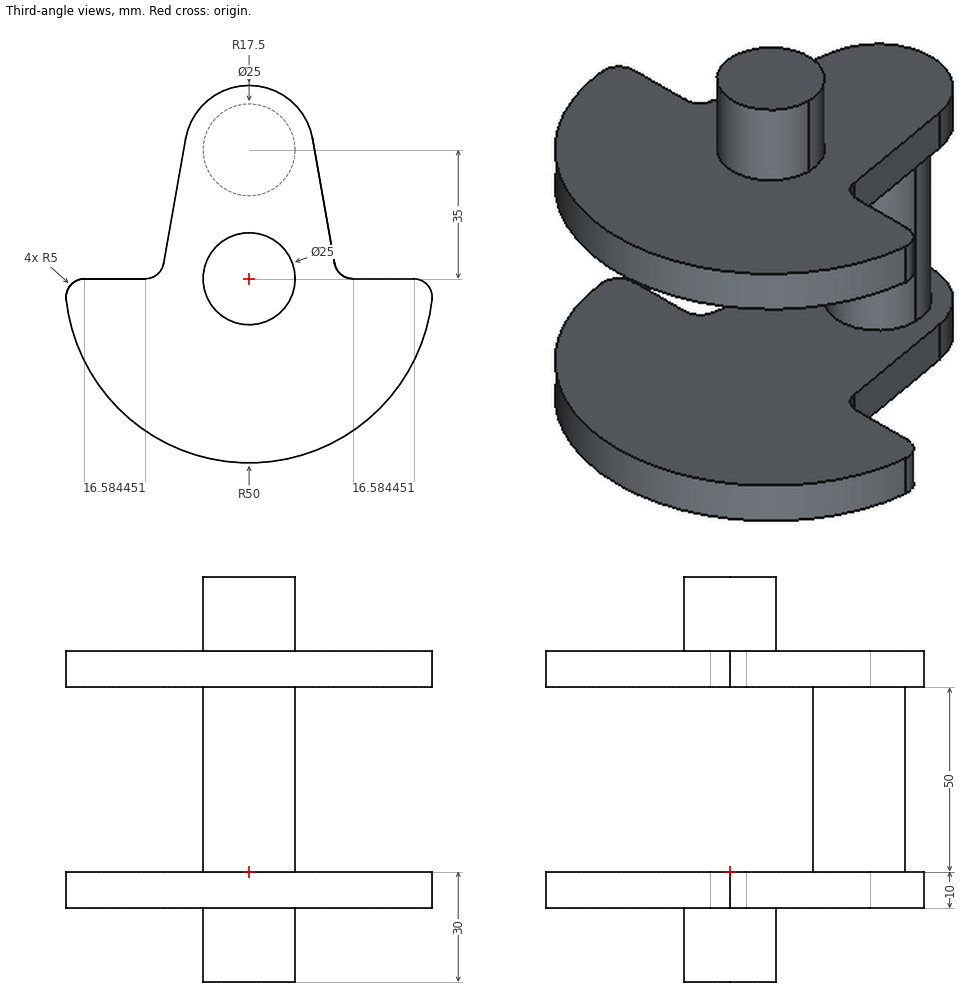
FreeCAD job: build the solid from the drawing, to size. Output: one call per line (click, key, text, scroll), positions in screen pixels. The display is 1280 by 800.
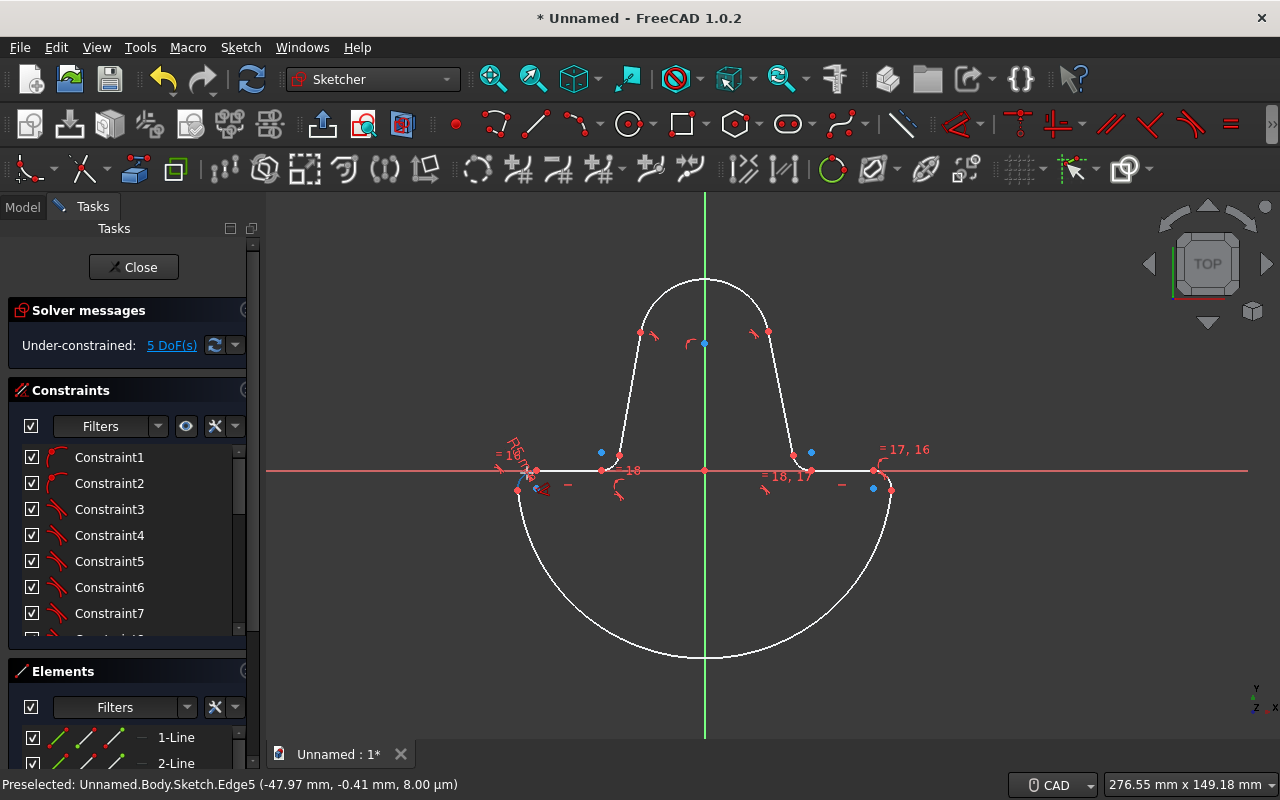
click(601, 627)
click(583, 654)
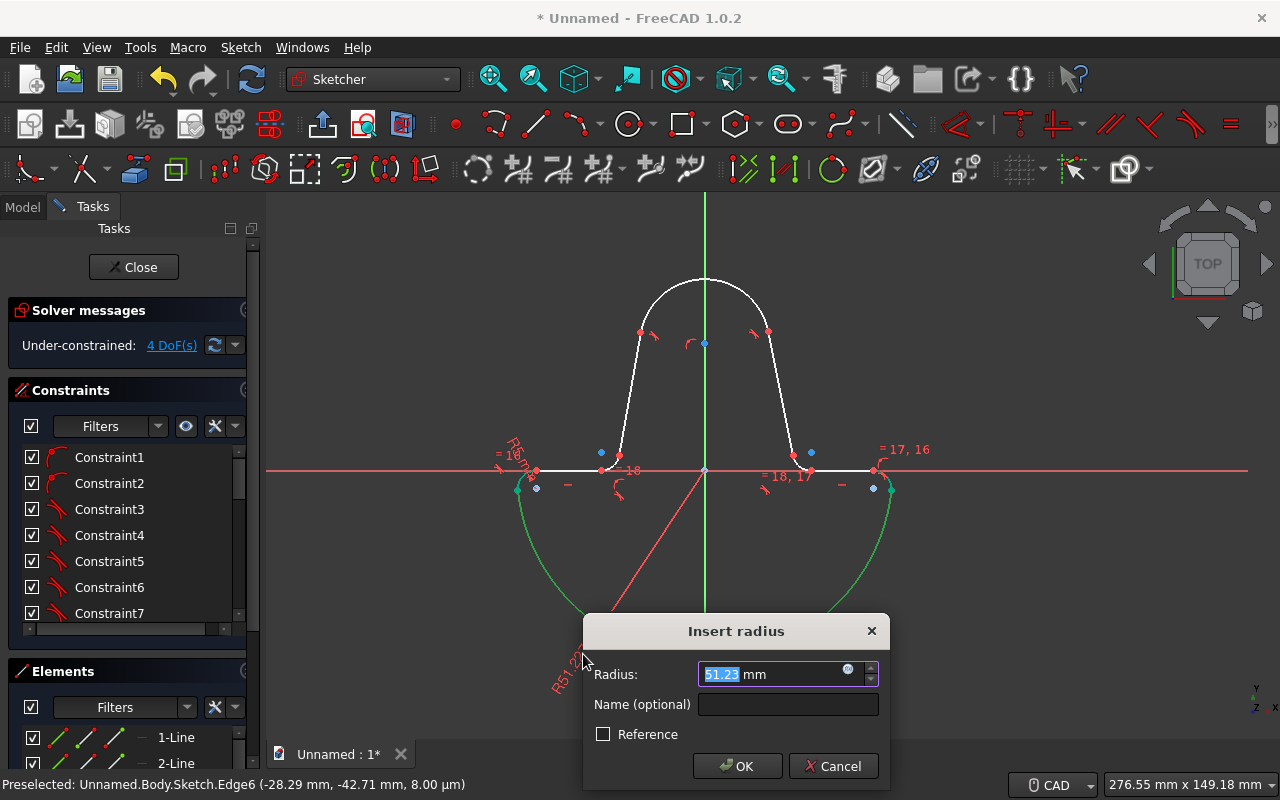
text(50)
key(Return)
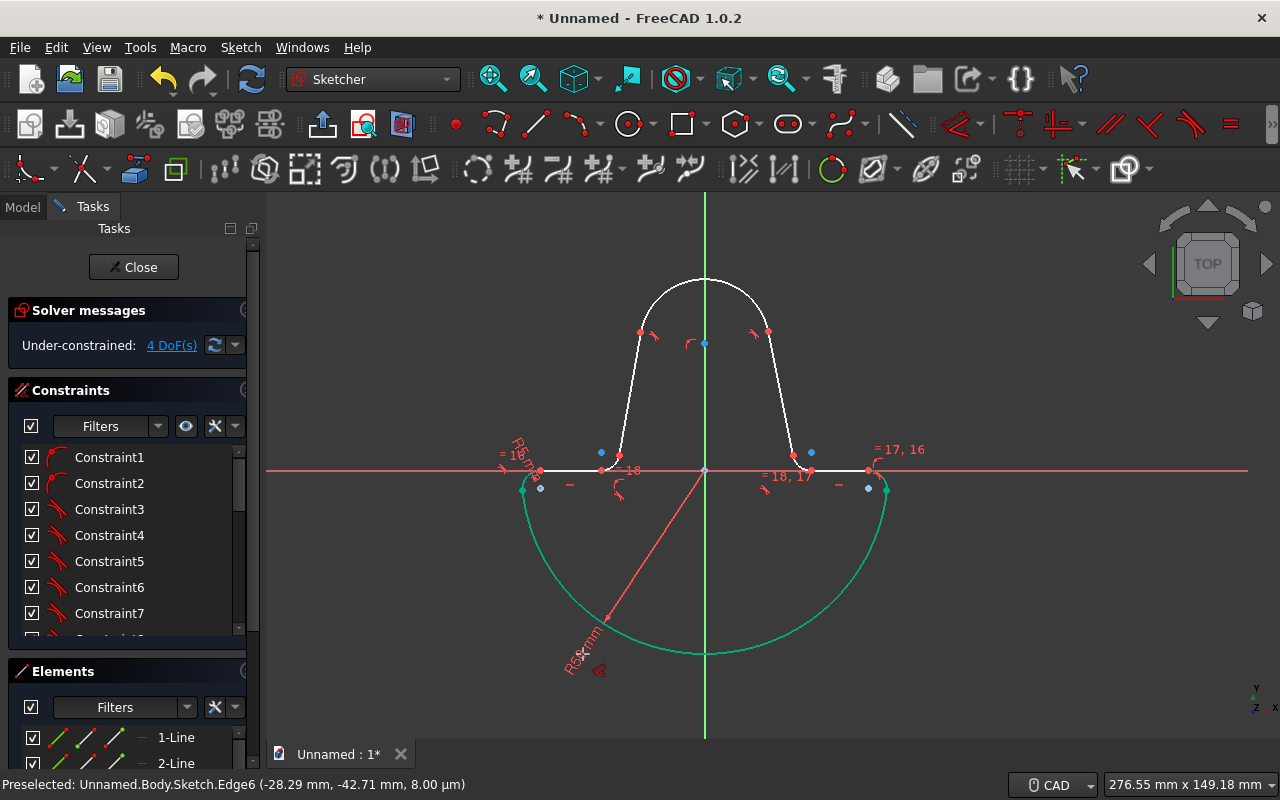
click(738, 289)
click(755, 262)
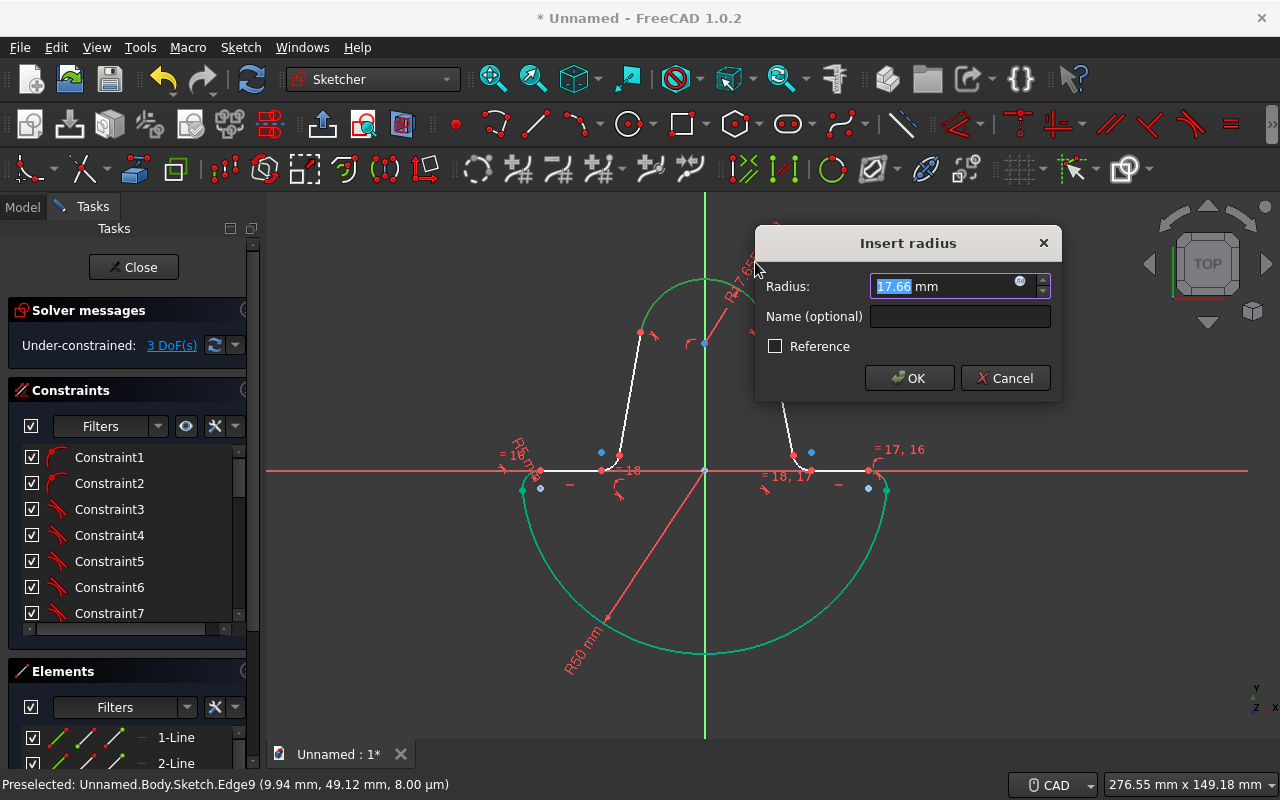
text(17.5)
key(Return)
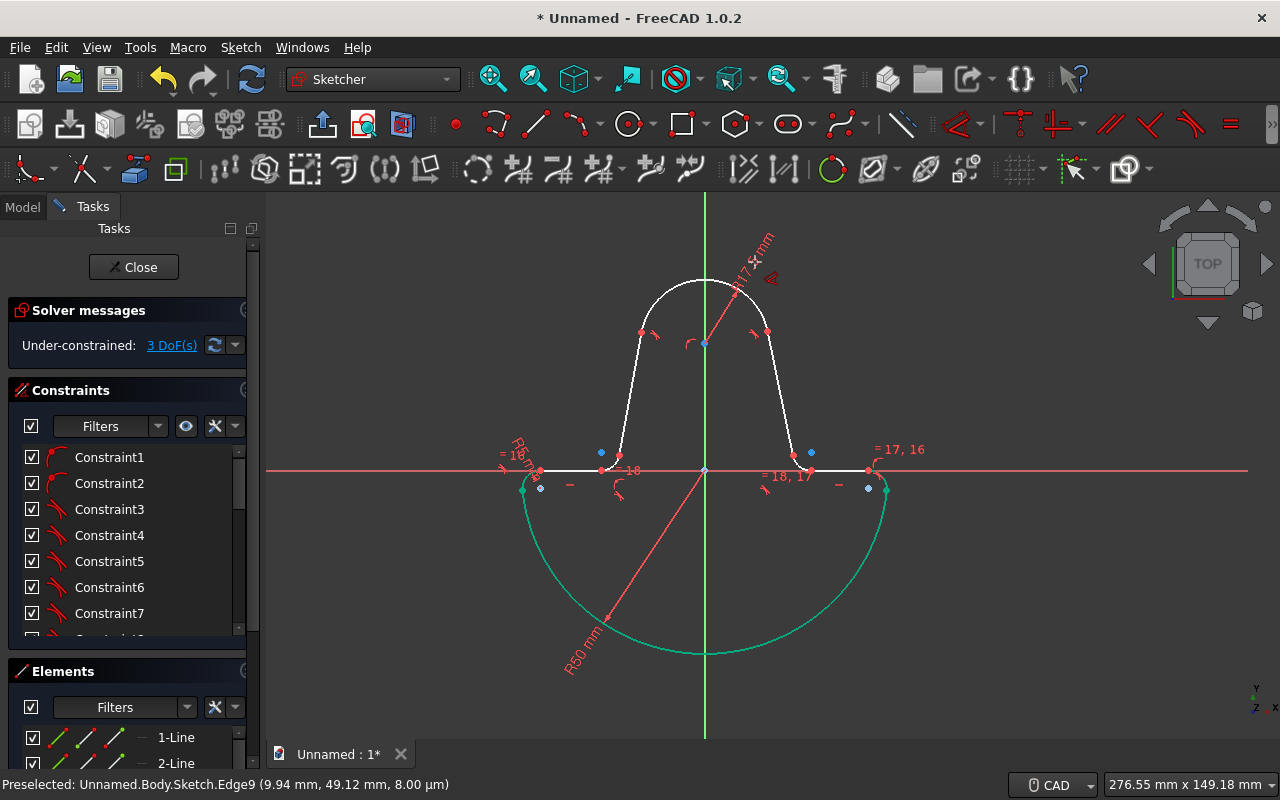
click(705, 344)
click(739, 407)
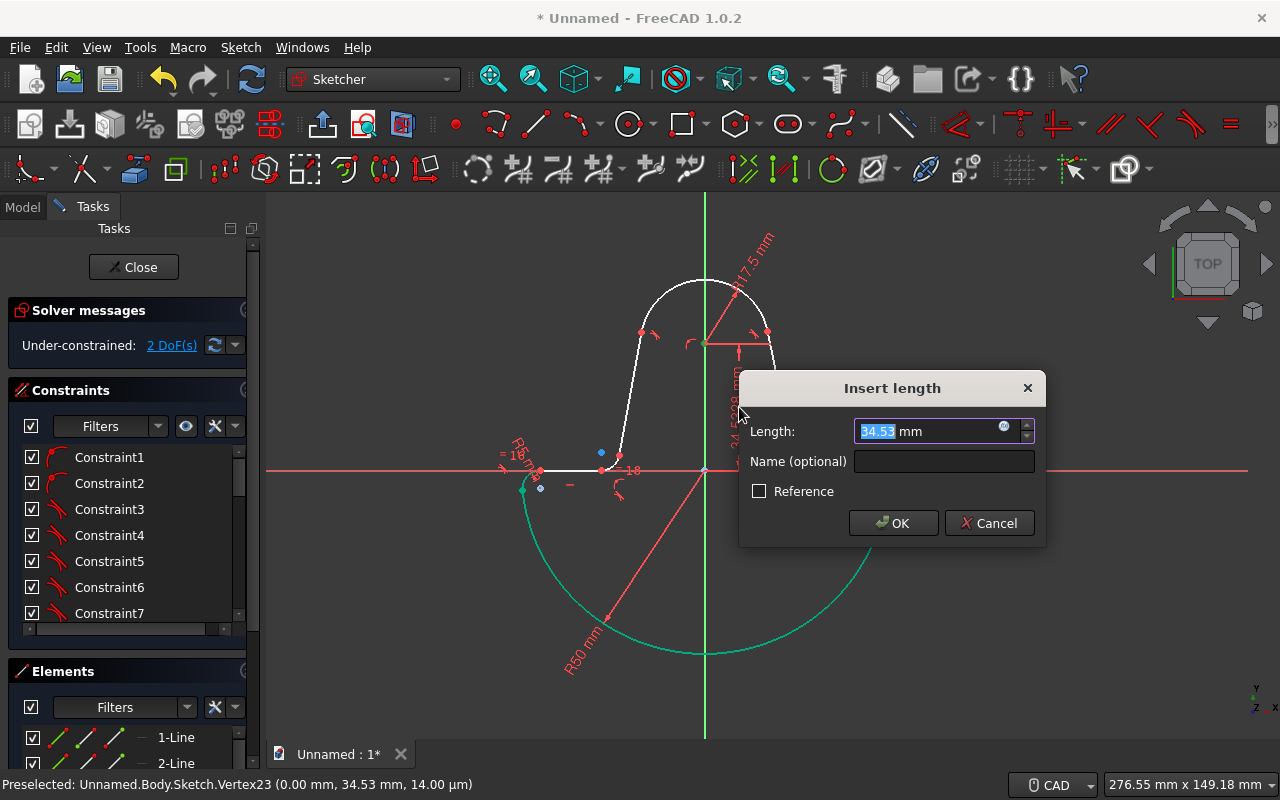
text(35)
key(Return)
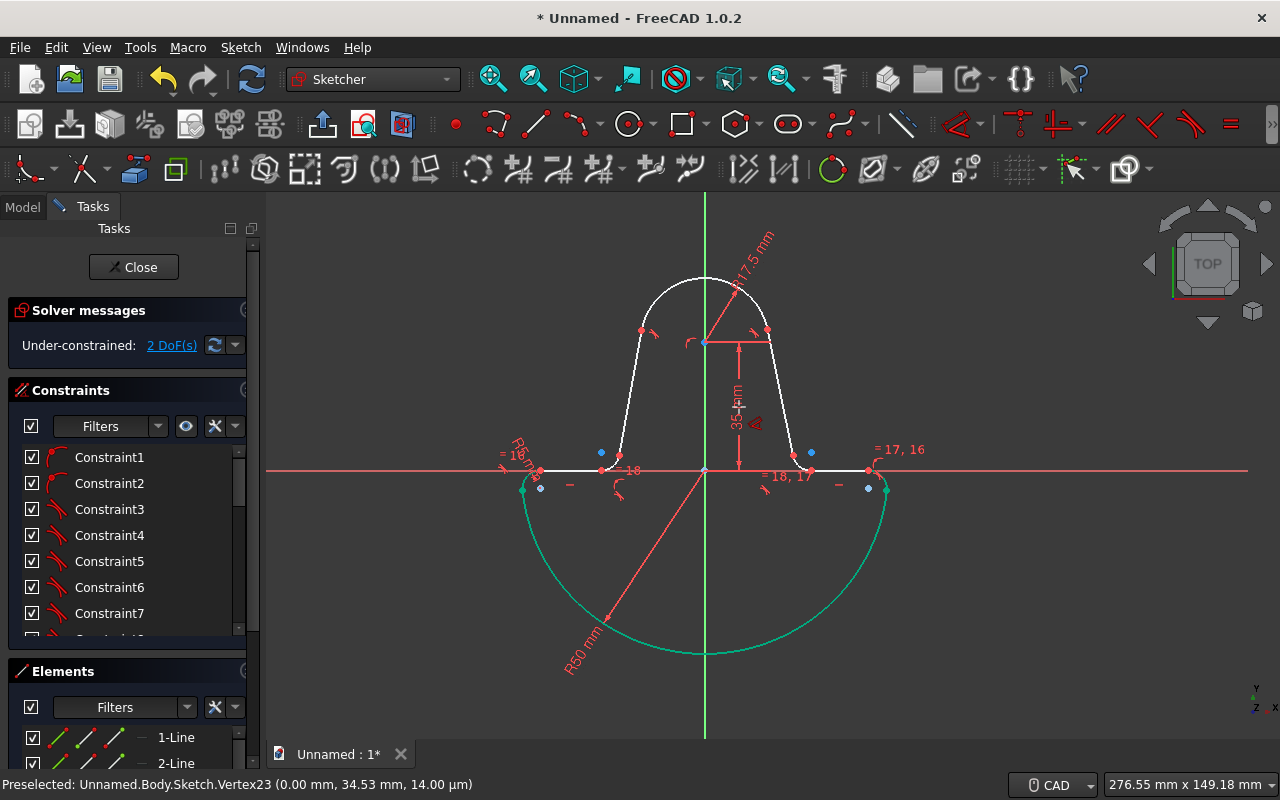
click(583, 471)
click(571, 505)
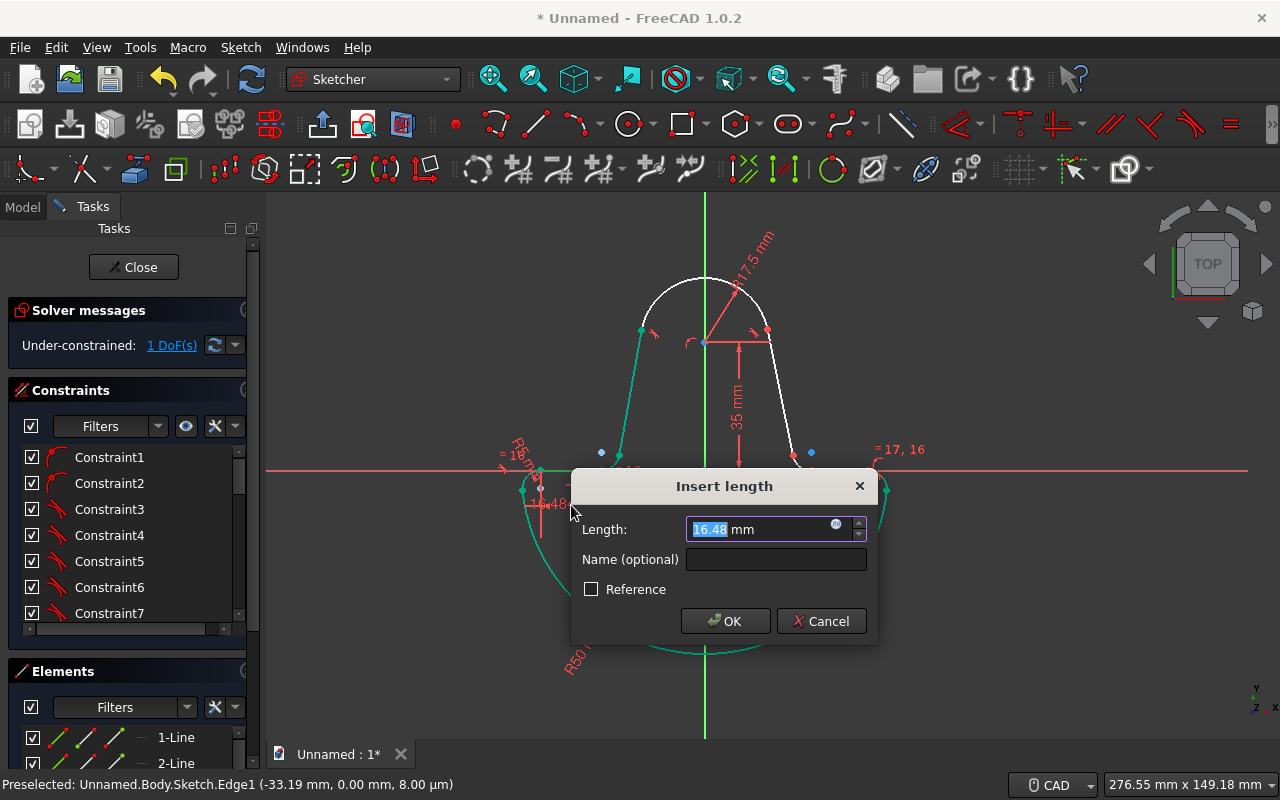
text(16.584451)
key(Return)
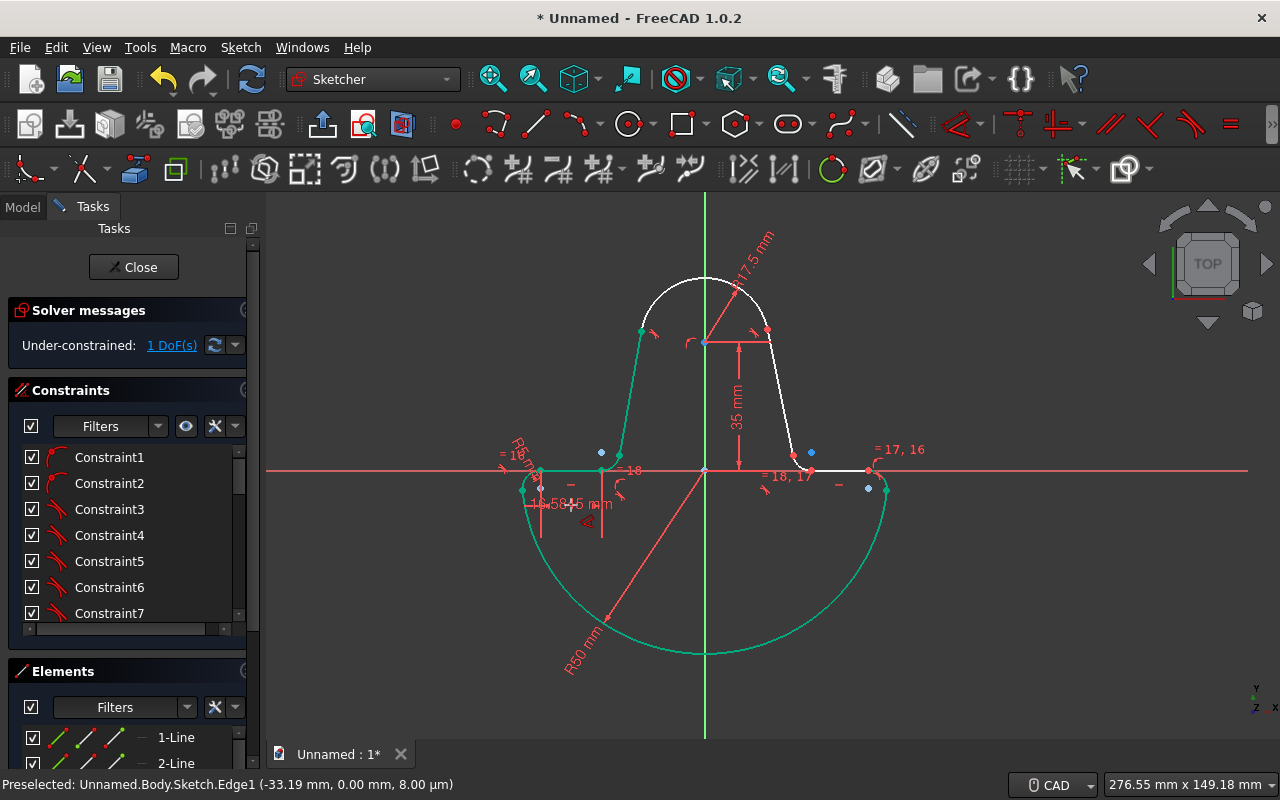
click(851, 471)
click(840, 505)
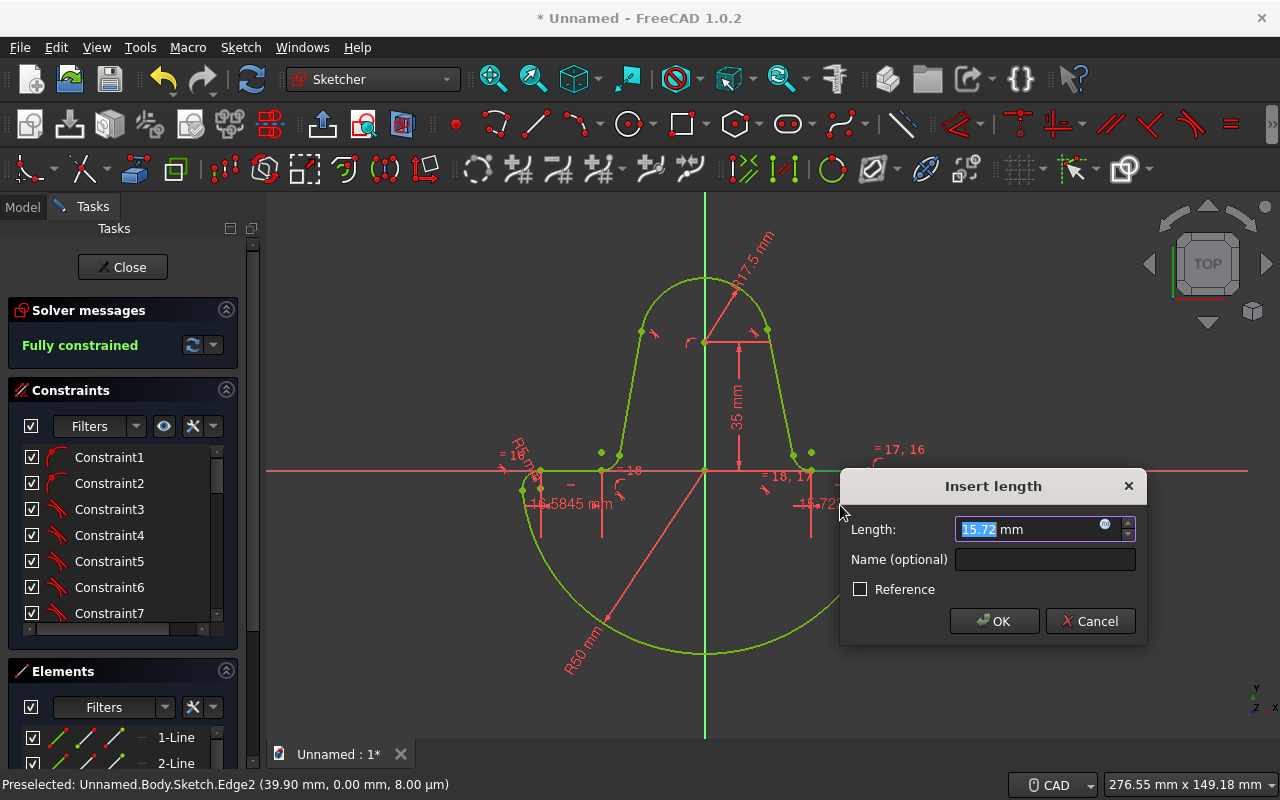
text(16.584451)
key(Return)
key(Escape)